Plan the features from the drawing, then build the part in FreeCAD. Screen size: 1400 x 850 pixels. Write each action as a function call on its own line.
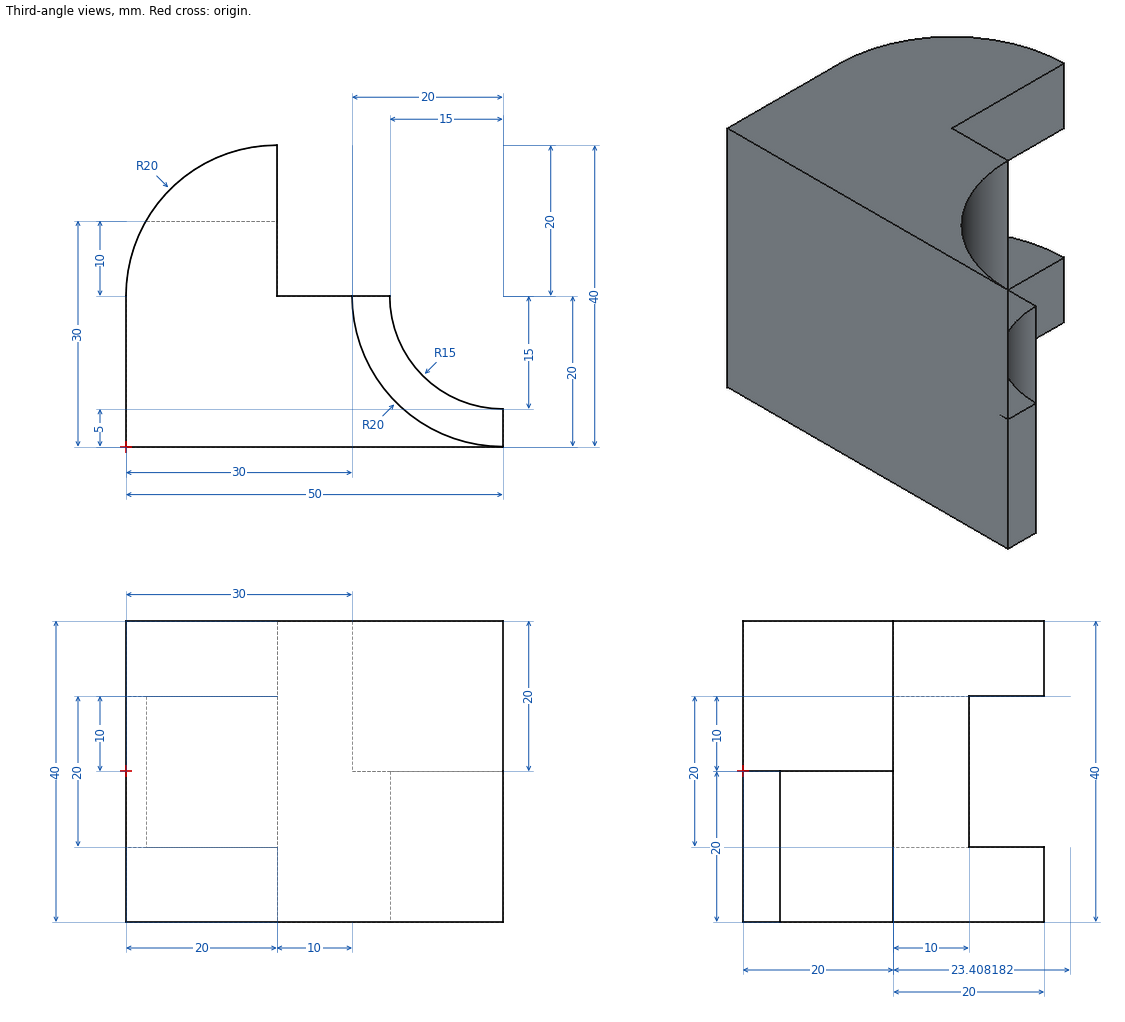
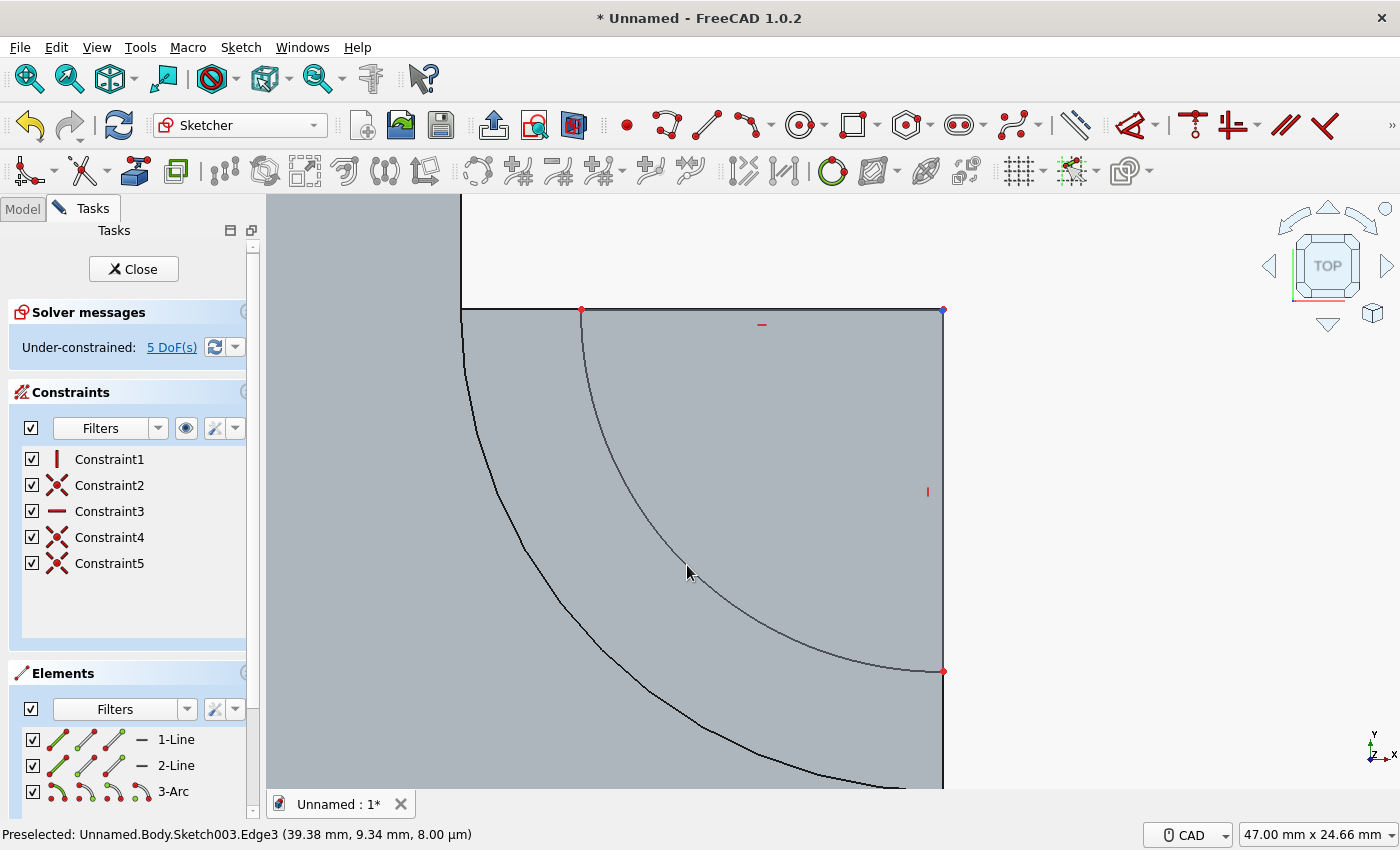
click(1130, 126)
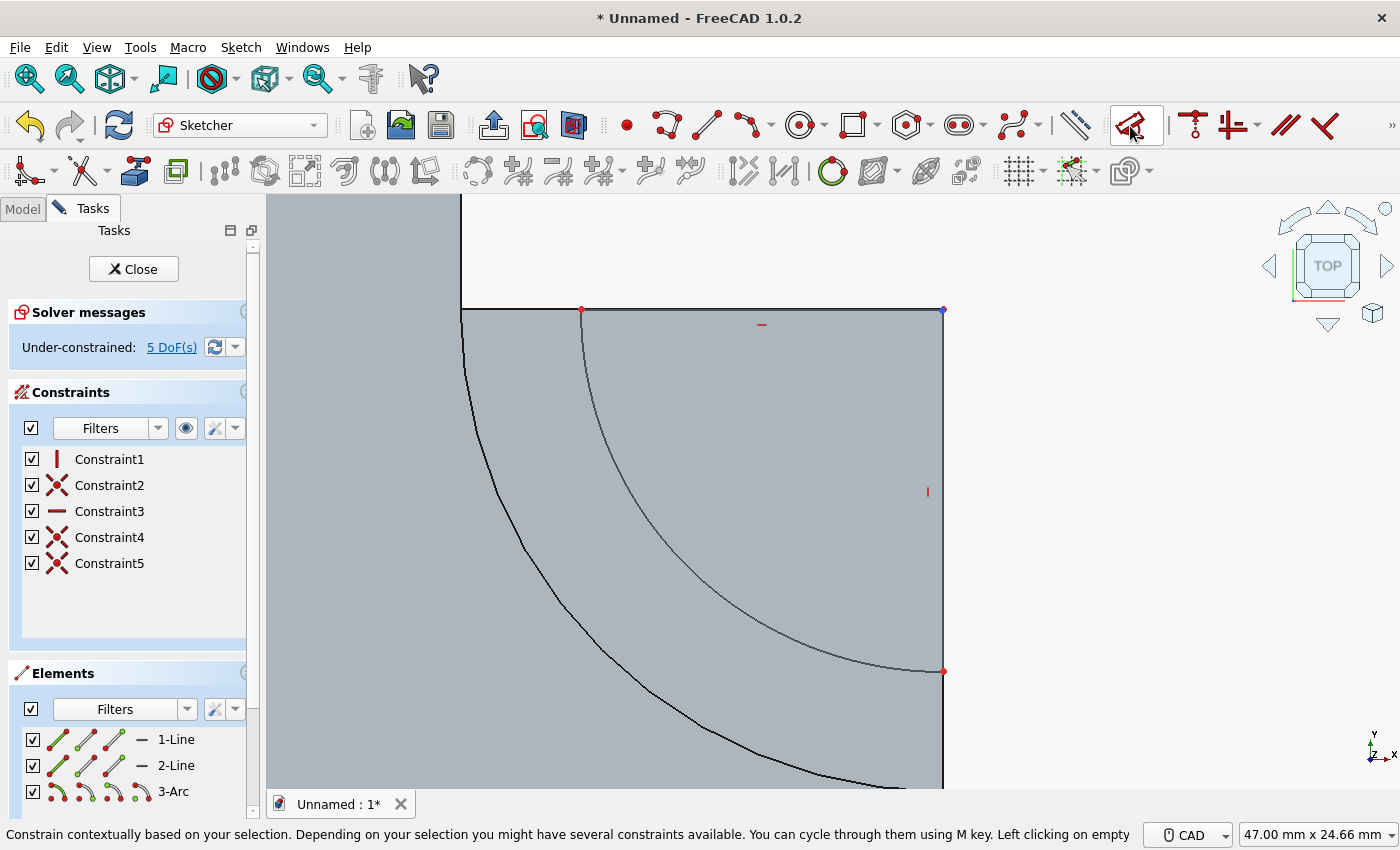
click(620, 474)
click(591, 488)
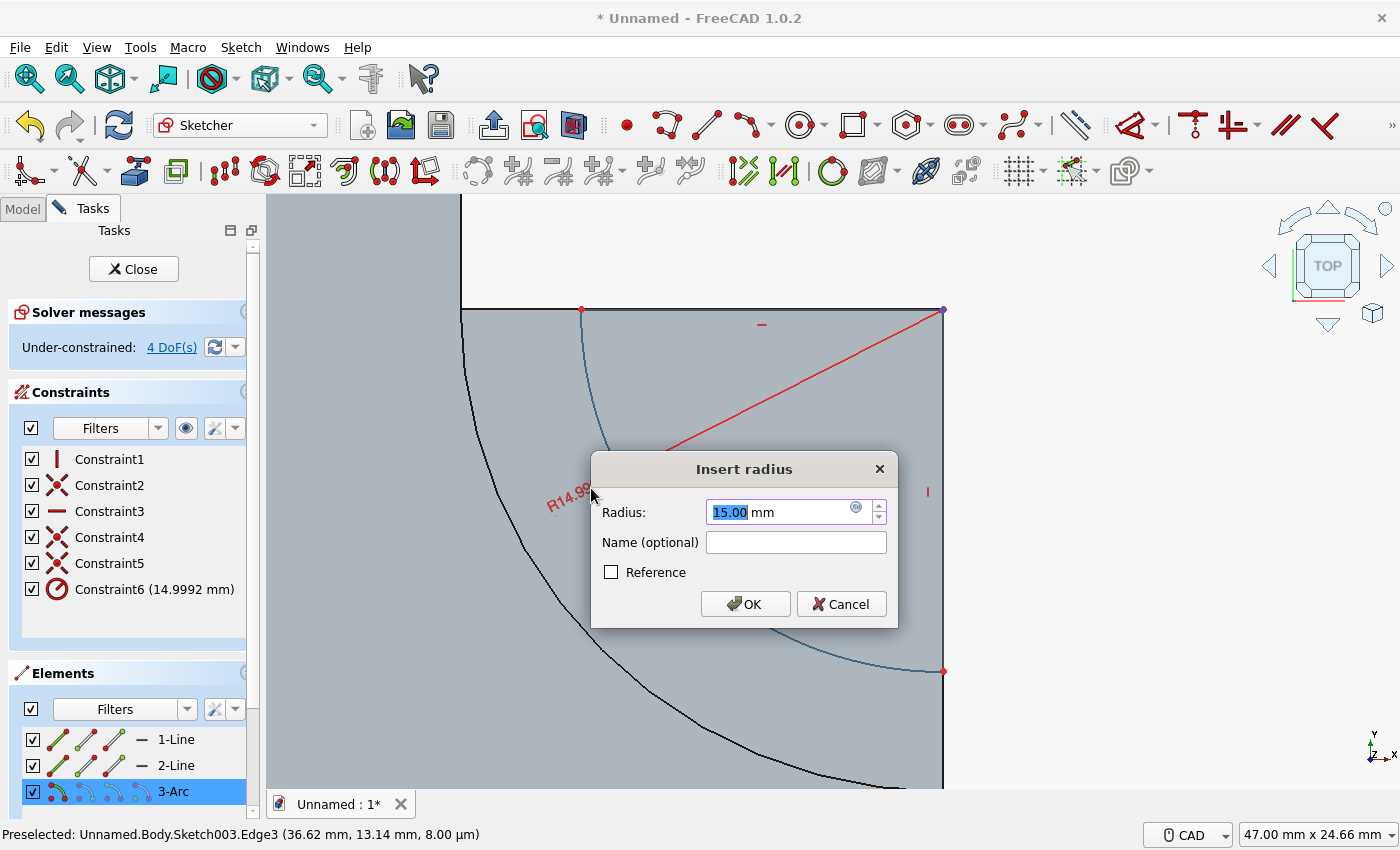
text(15)
key(Return)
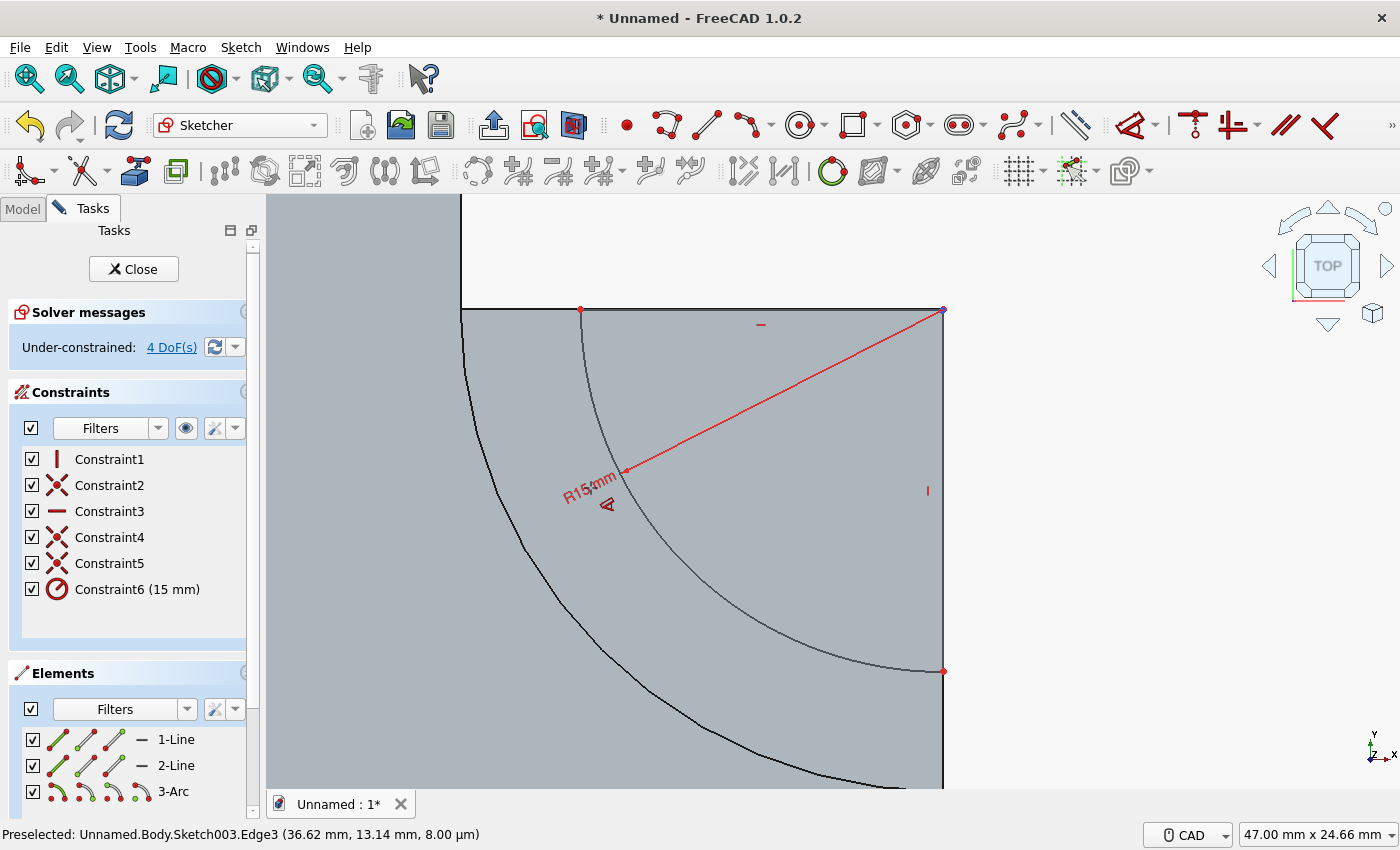
click(943, 563)
click(977, 491)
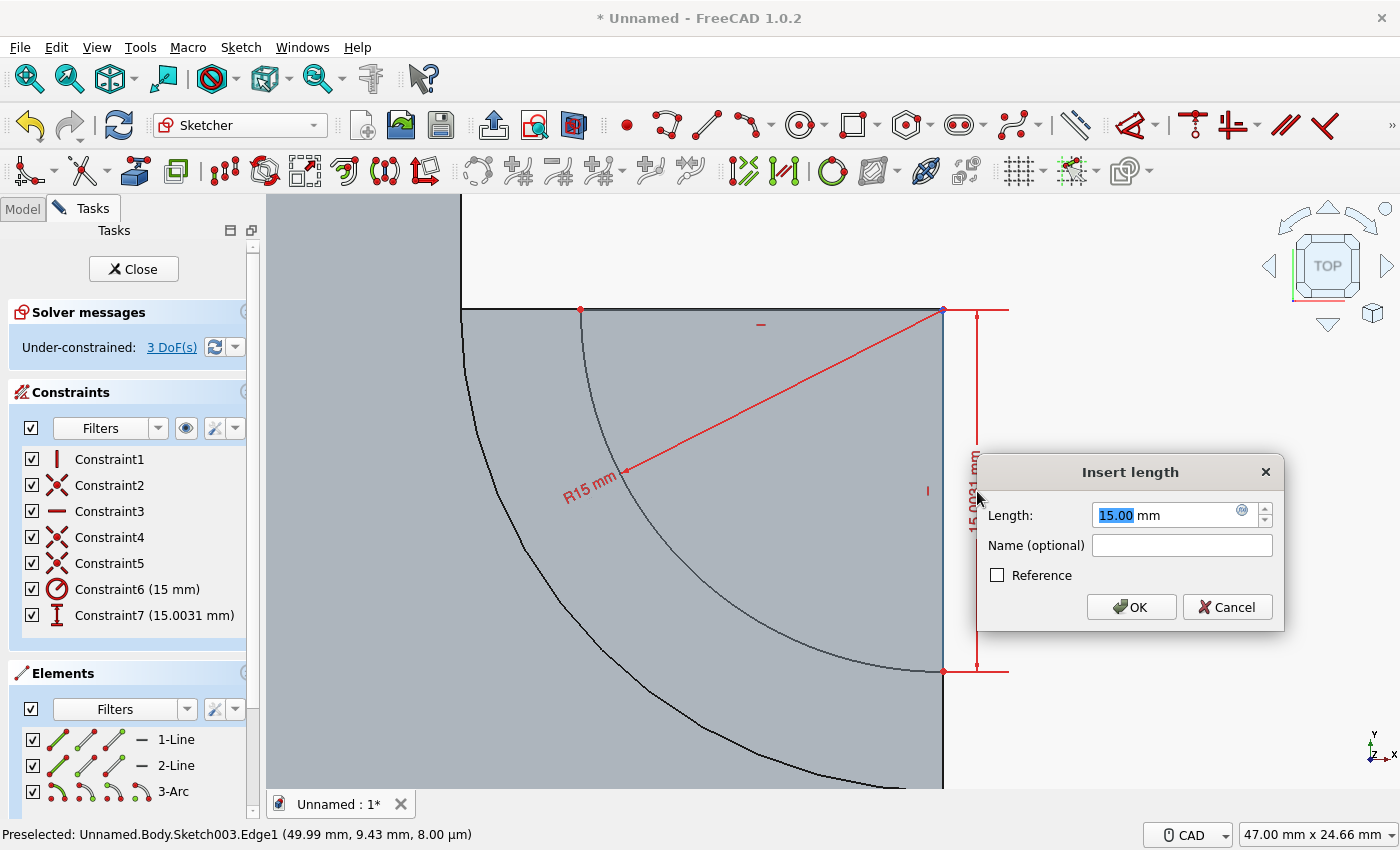
text(15)
key(Return)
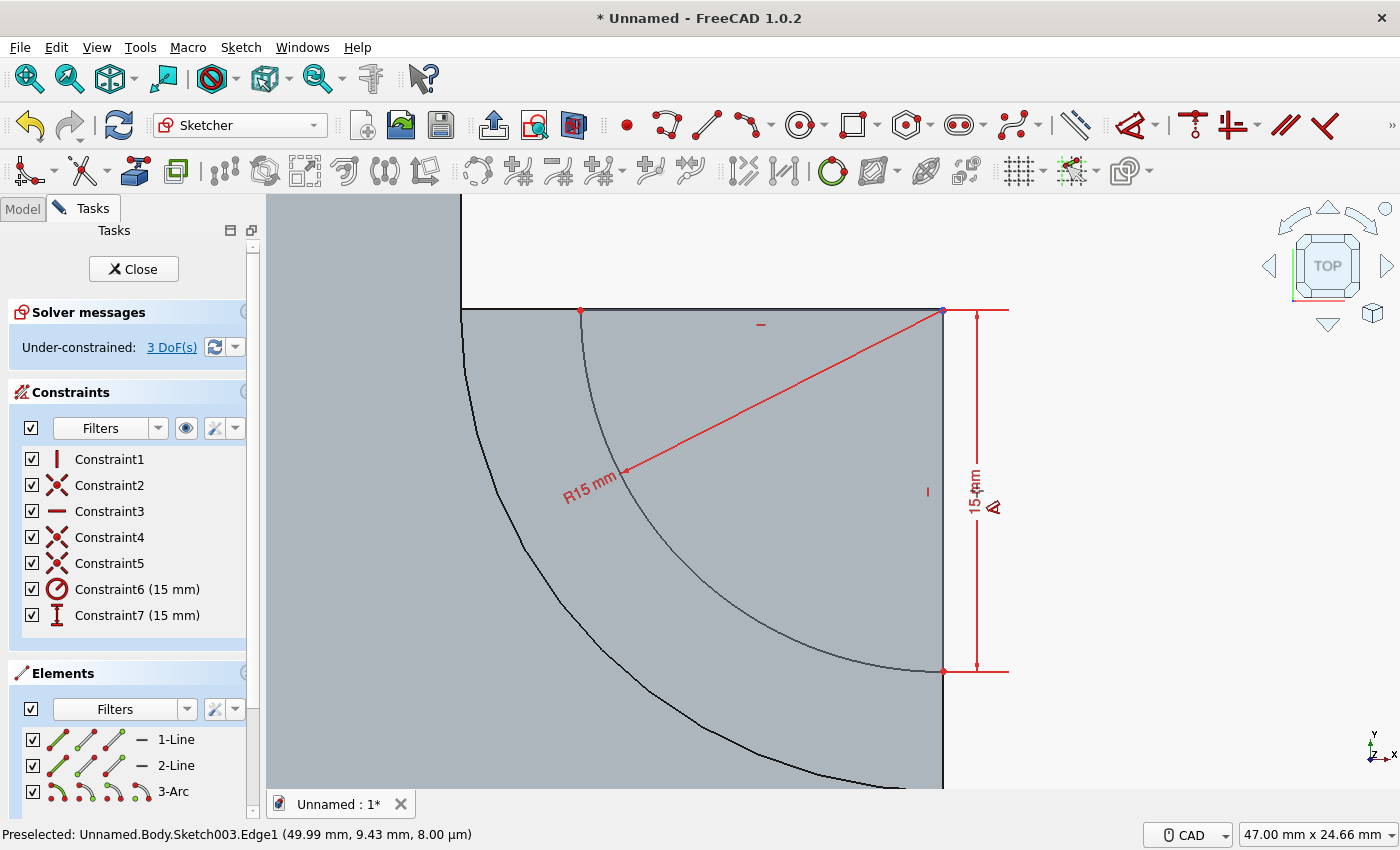
click(834, 310)
click(762, 276)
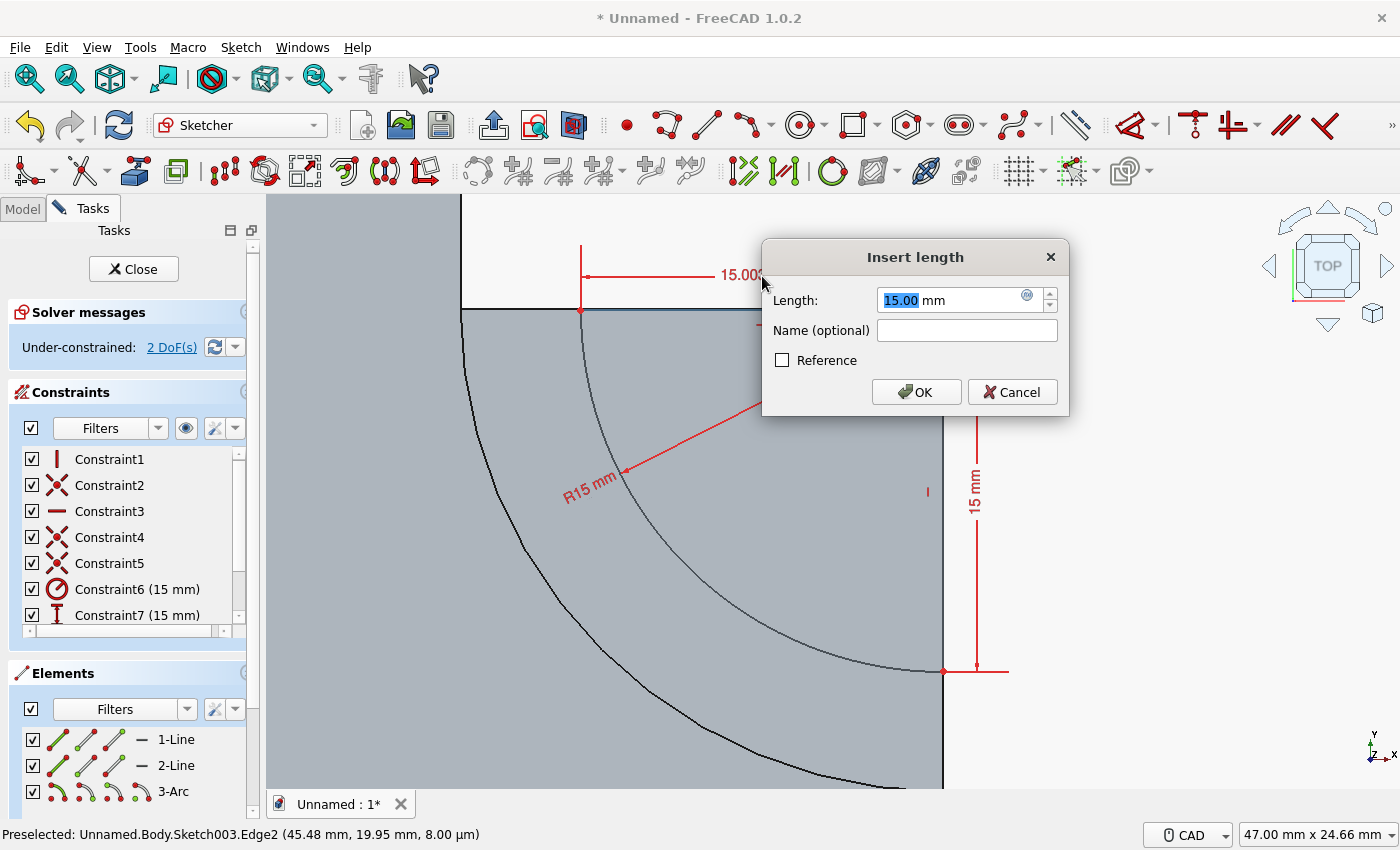
text(15)
key(Return)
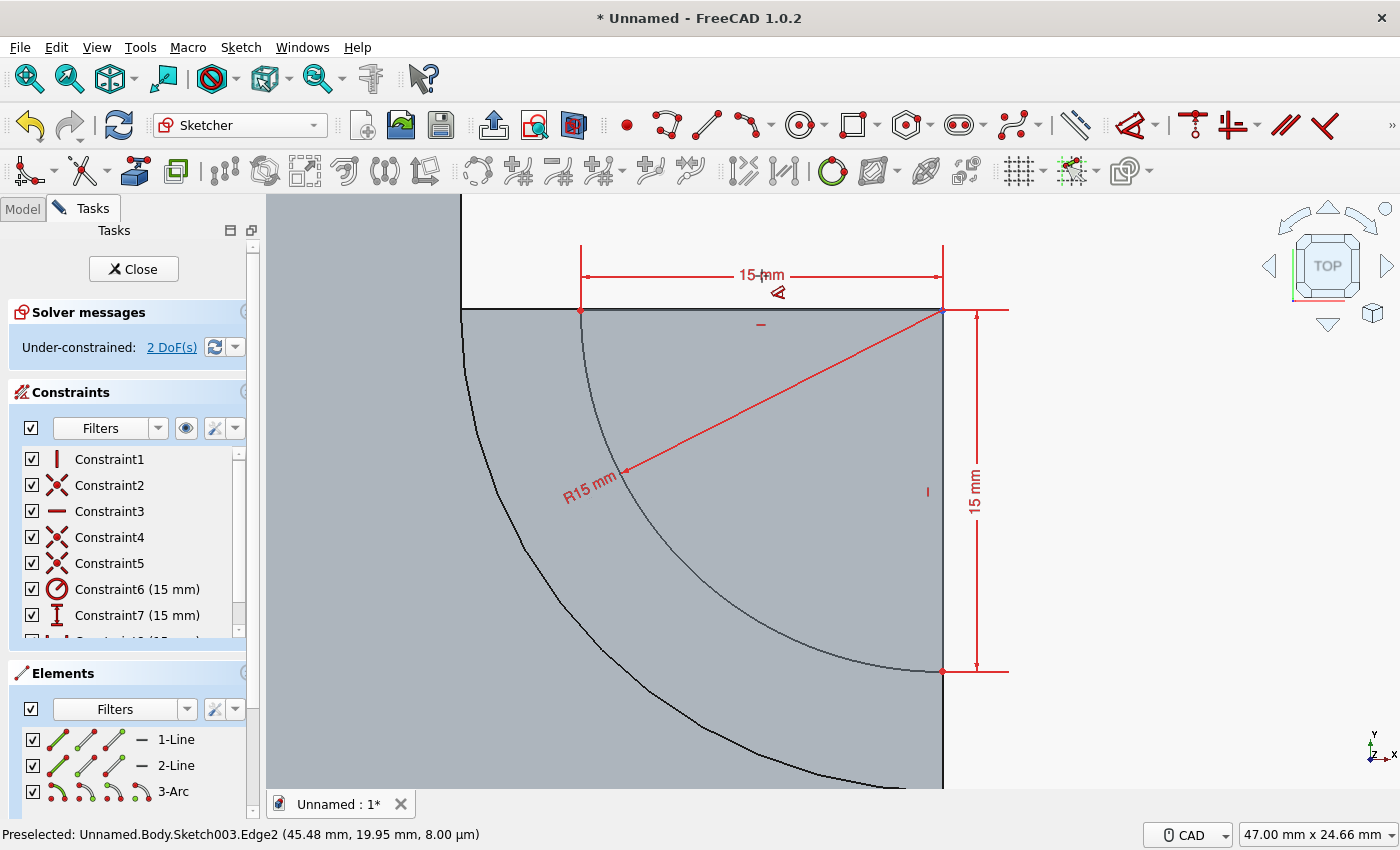
click(943, 672)
click(977, 717)